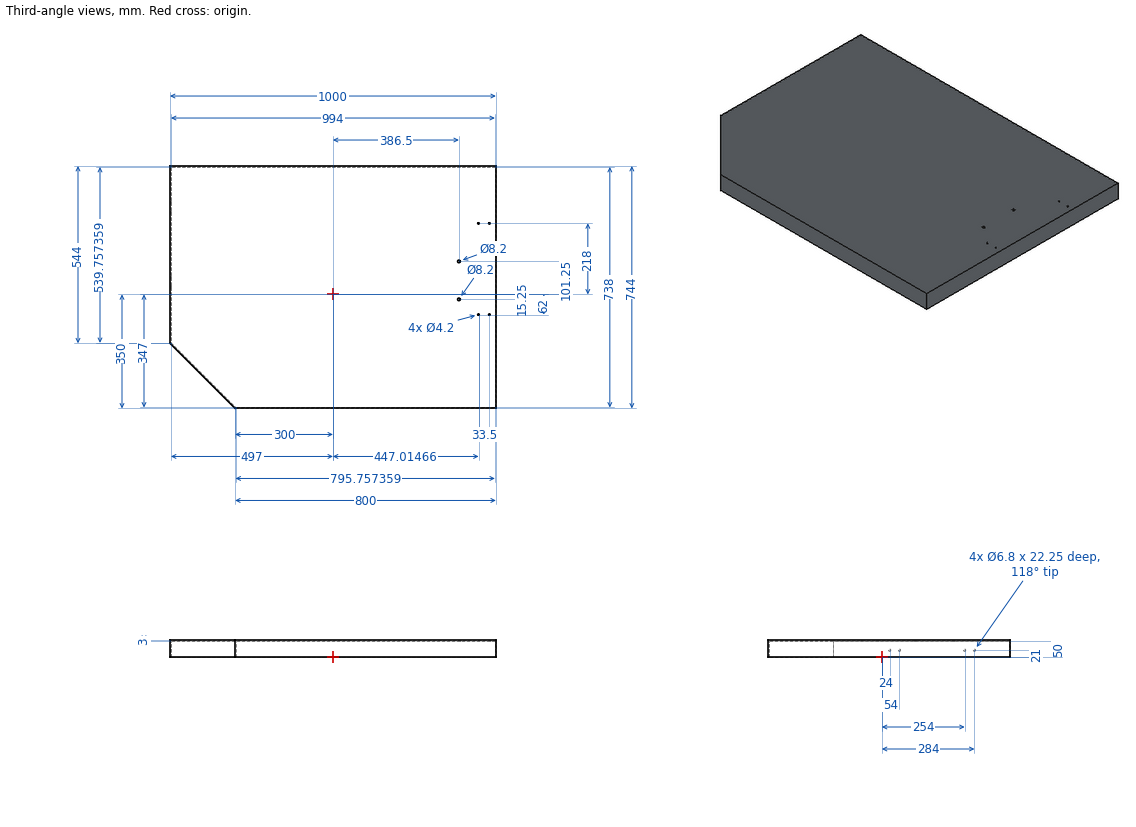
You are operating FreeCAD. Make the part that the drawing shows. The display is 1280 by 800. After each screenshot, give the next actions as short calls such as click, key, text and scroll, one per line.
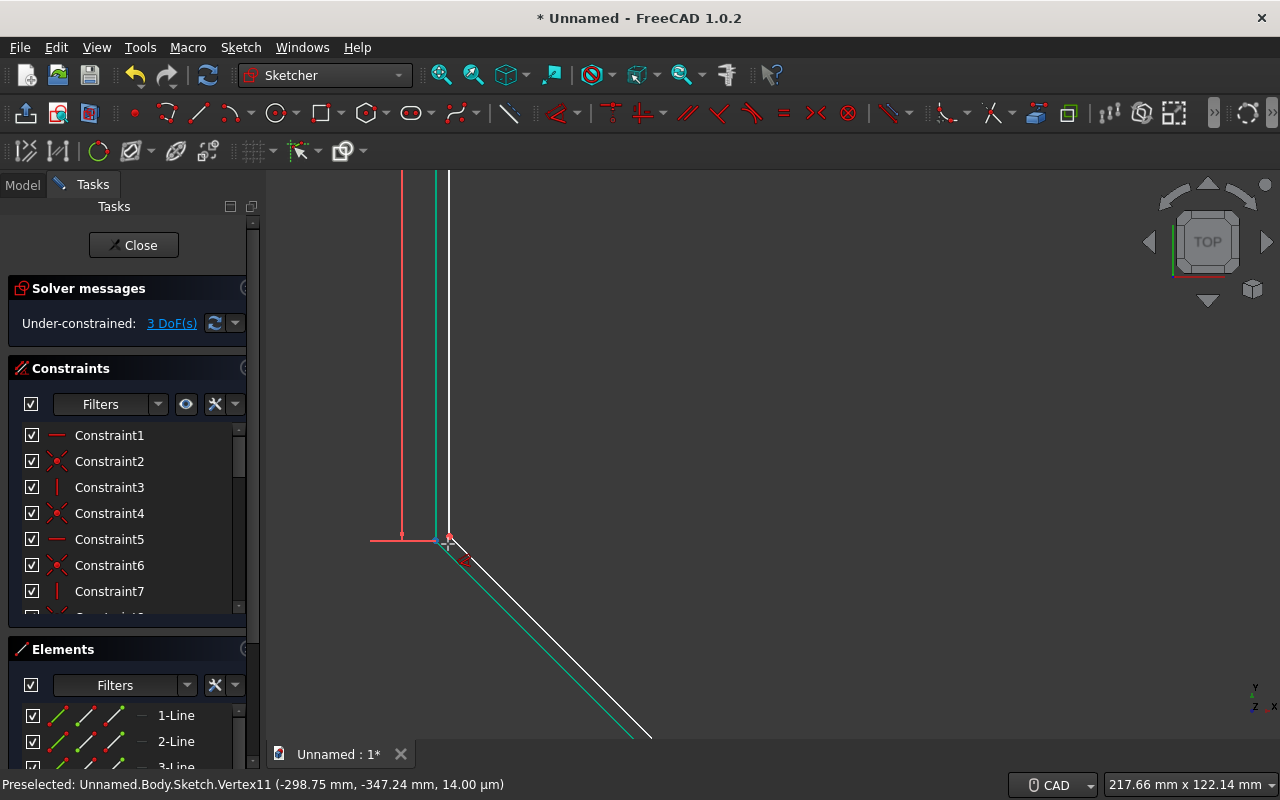
click(449, 536)
click(782, 570)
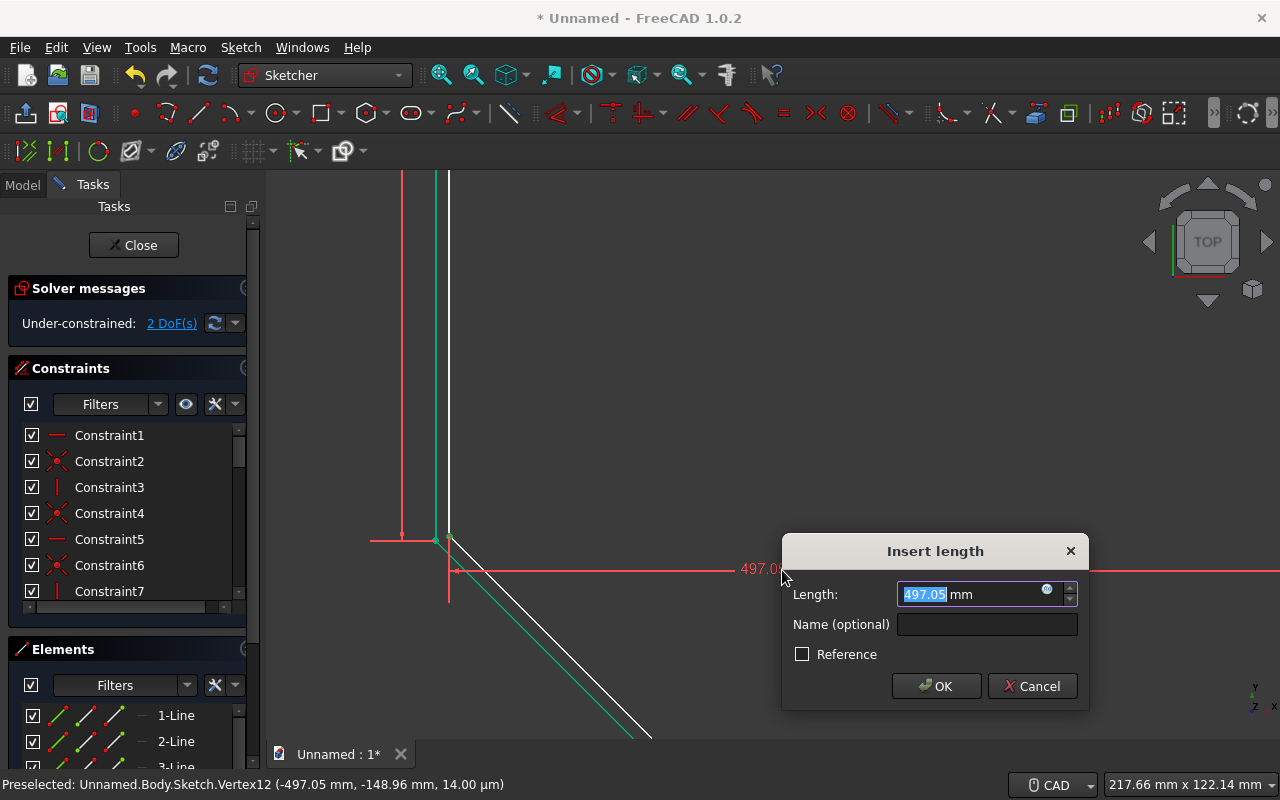
text(497)
key(Return)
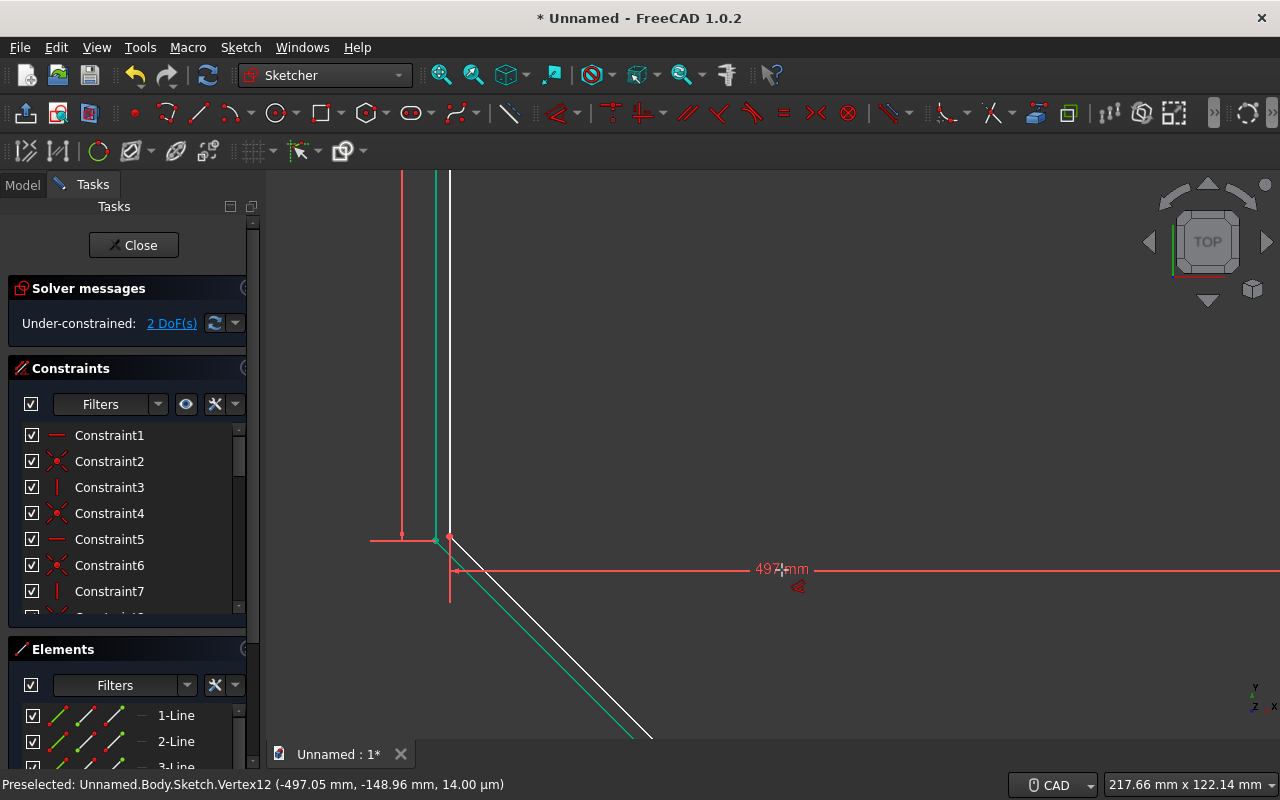
scroll(448, 544, down, 11)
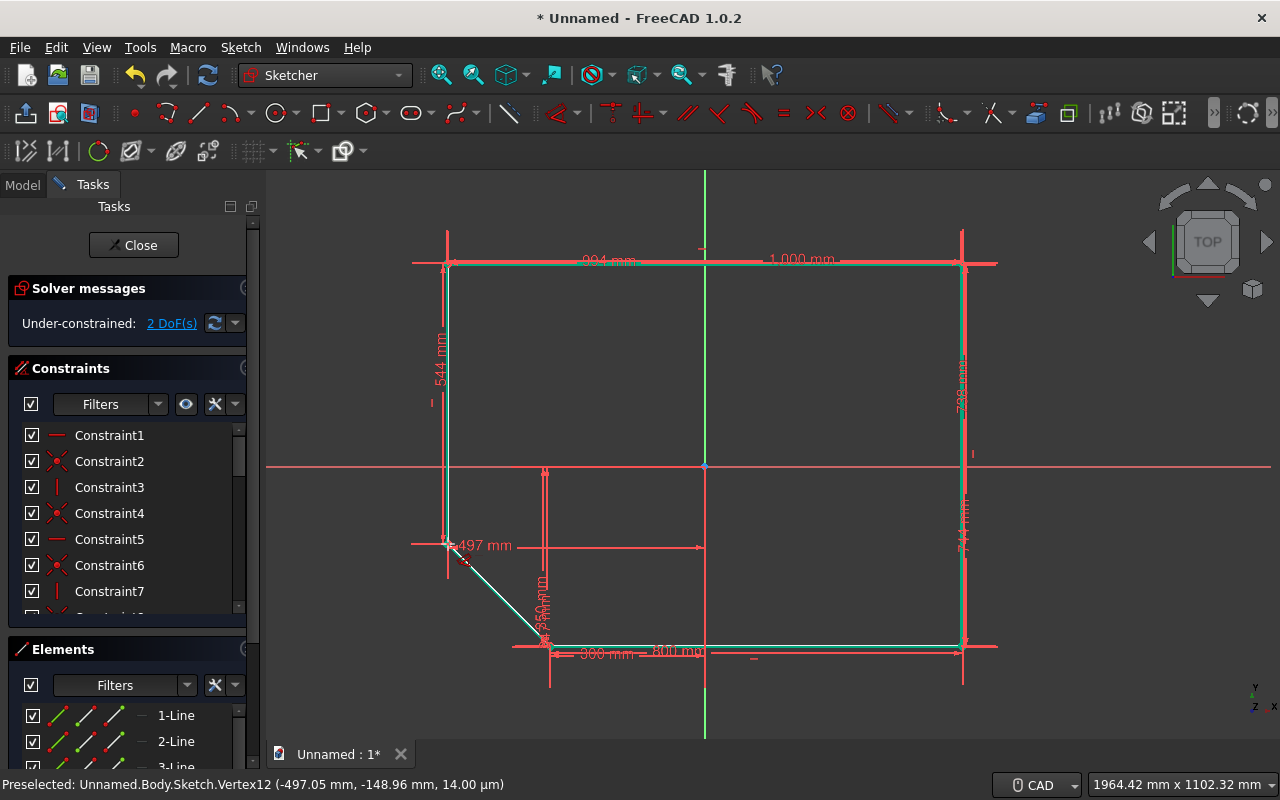
scroll(448, 460, up, 11)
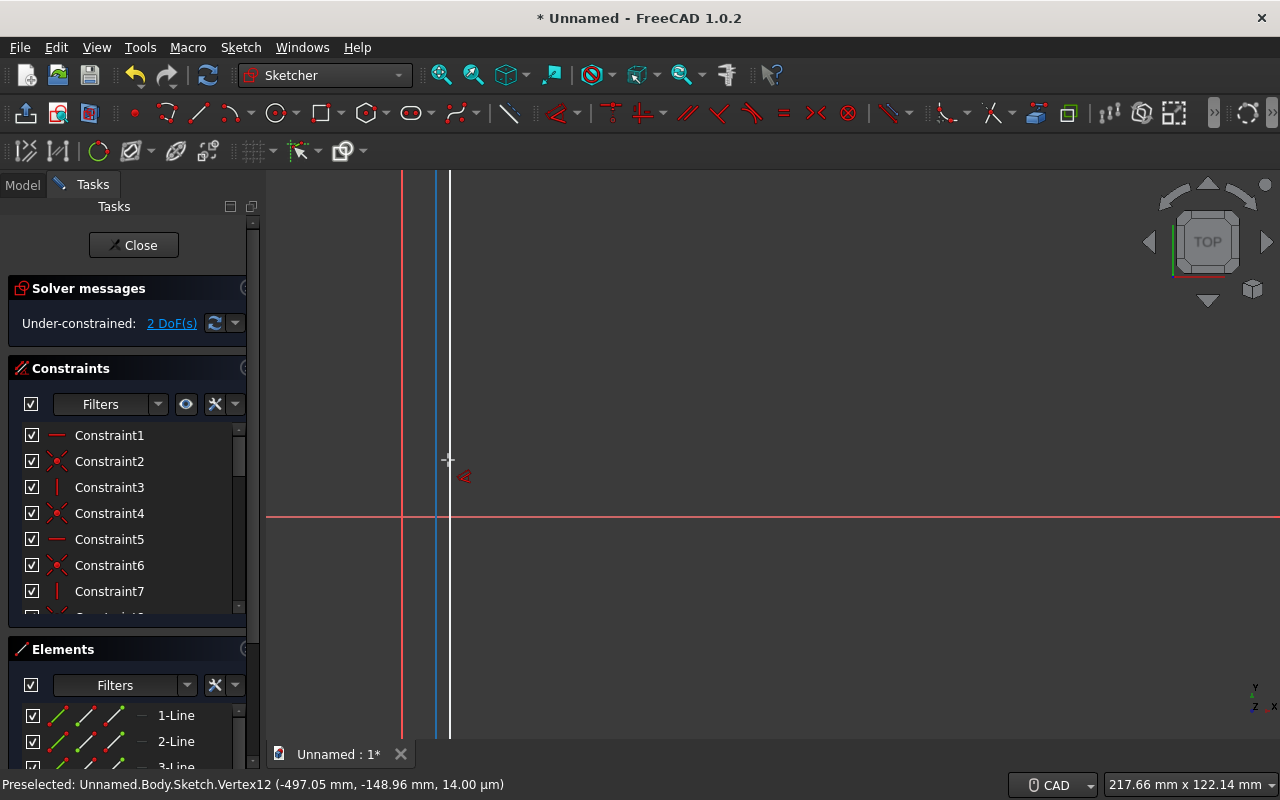
click(450, 457)
click(416, 454)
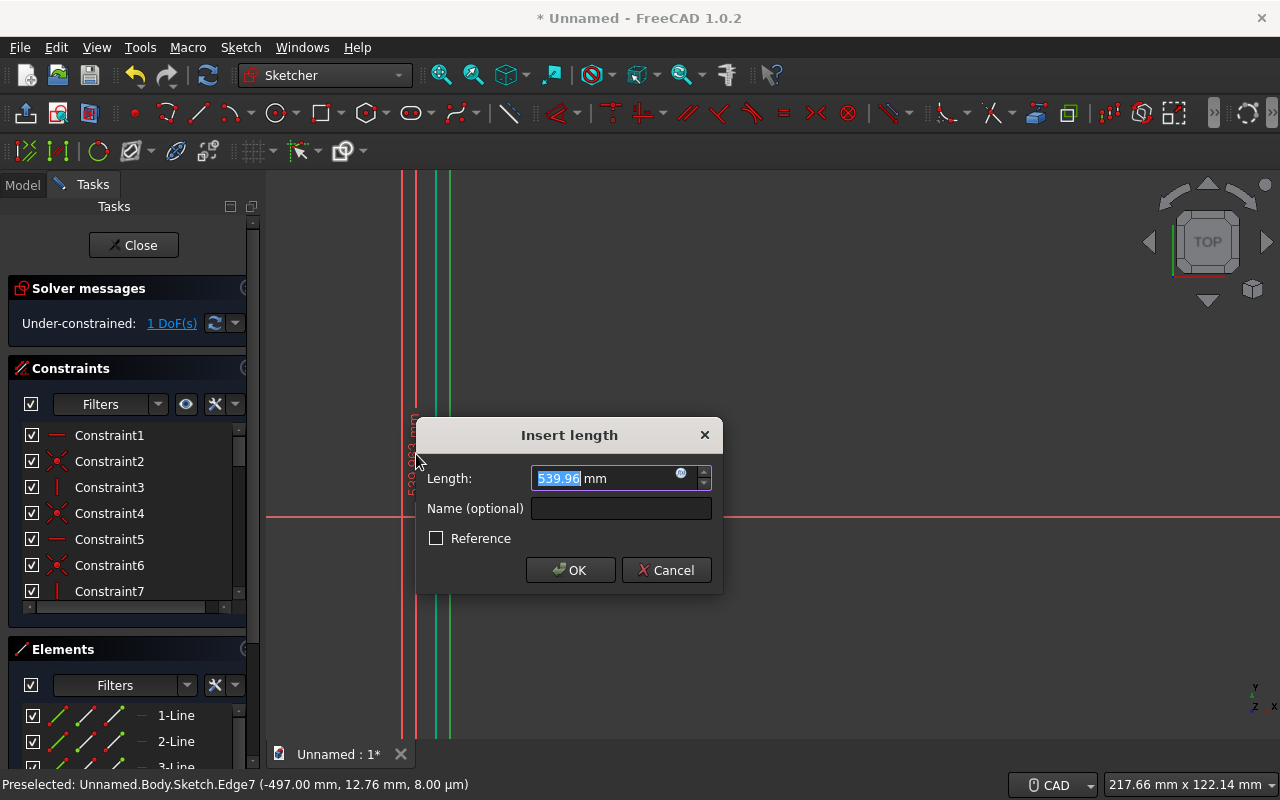
text(539.757359)
key(Return)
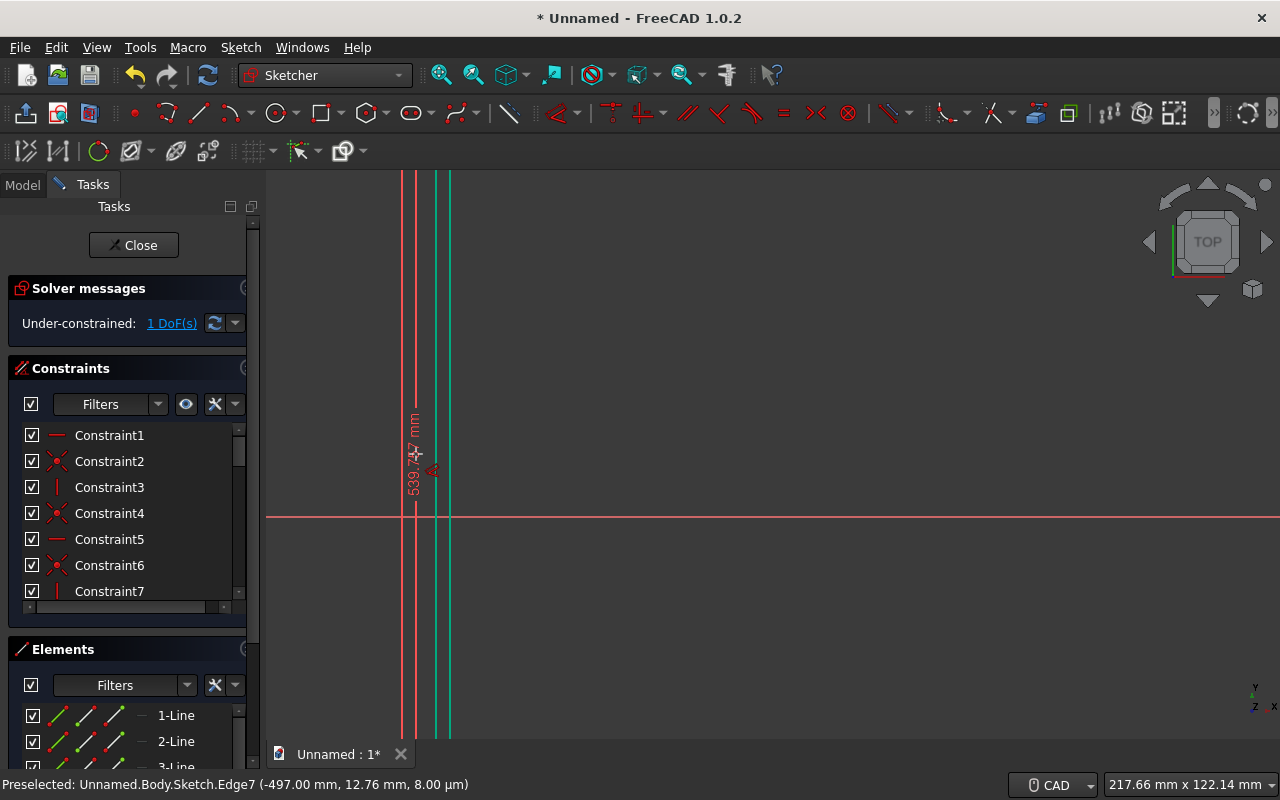
scroll(448, 459, down, 11)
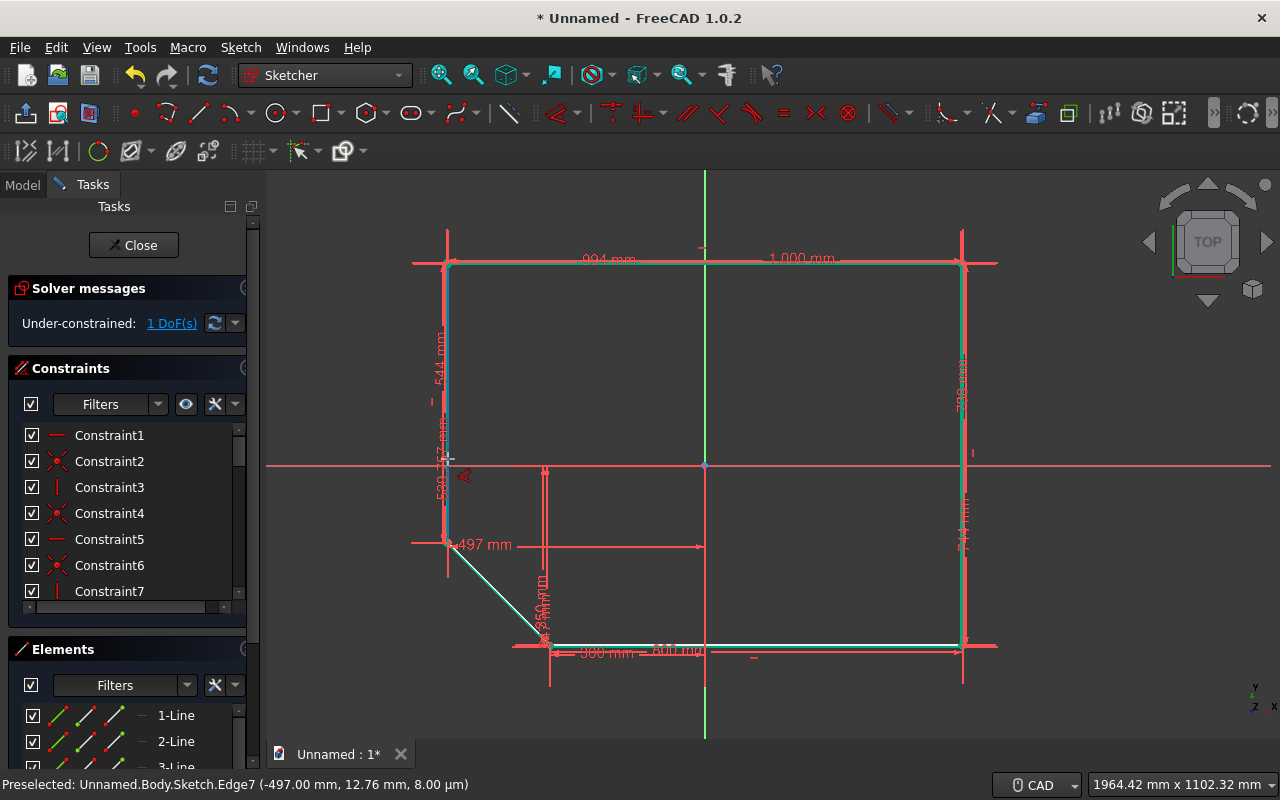
scroll(838, 645, up, 11)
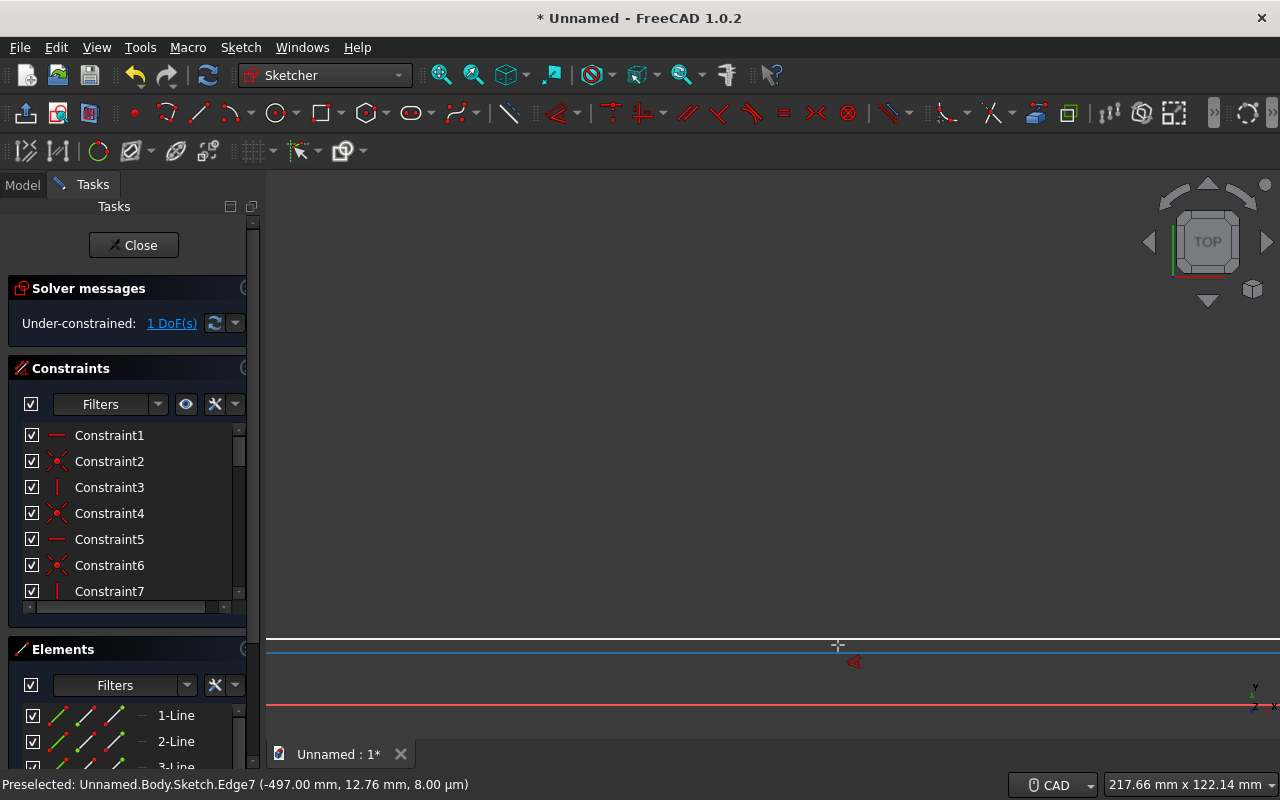
click(835, 639)
click(704, 673)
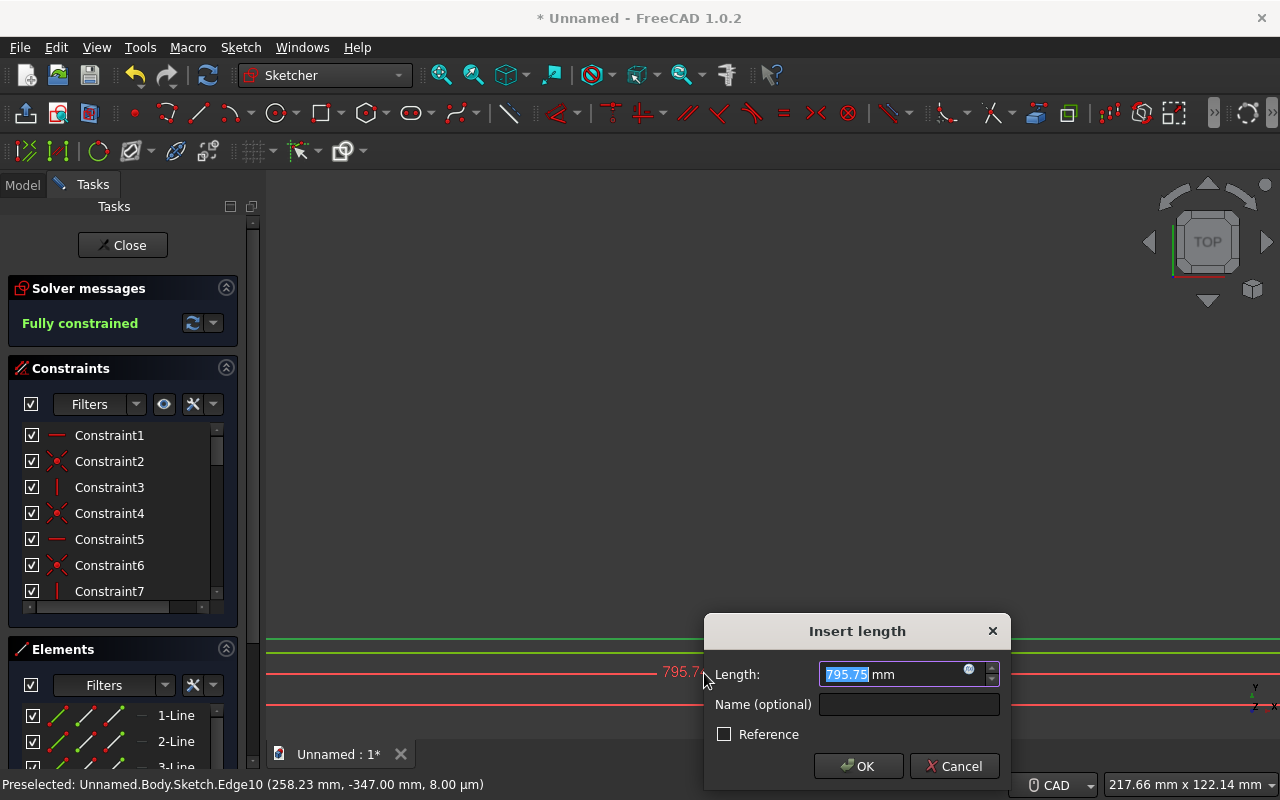
text(795.757359)
key(Return)
key(Escape)